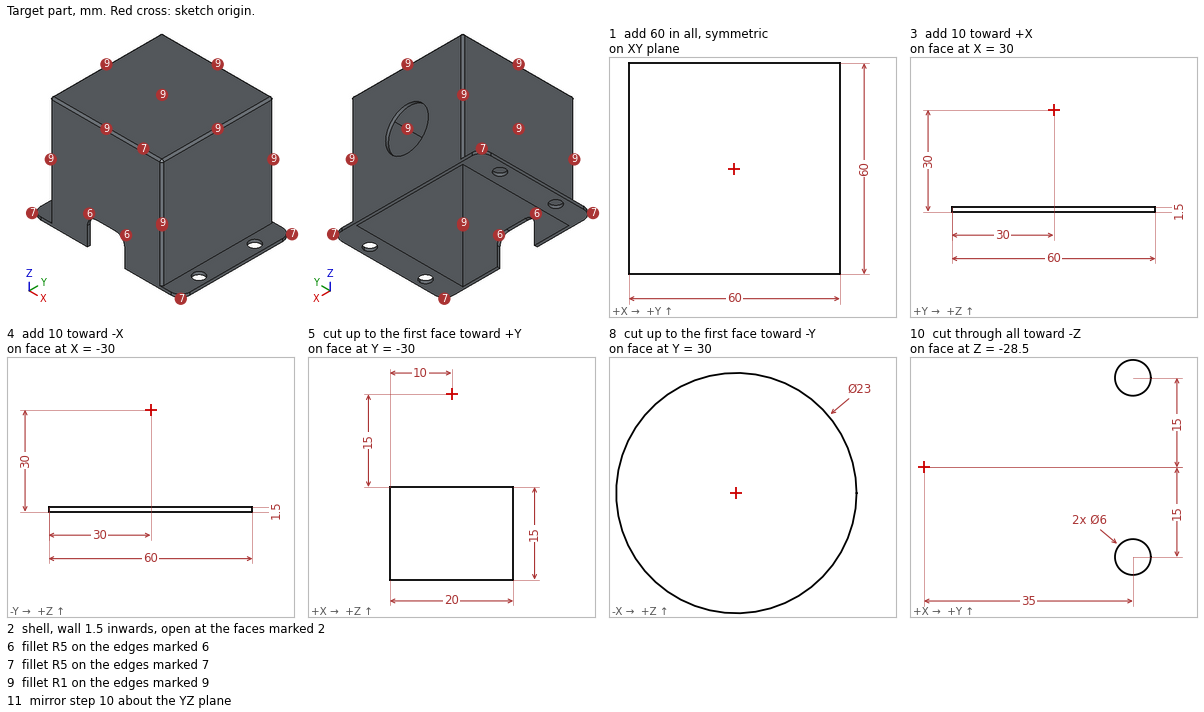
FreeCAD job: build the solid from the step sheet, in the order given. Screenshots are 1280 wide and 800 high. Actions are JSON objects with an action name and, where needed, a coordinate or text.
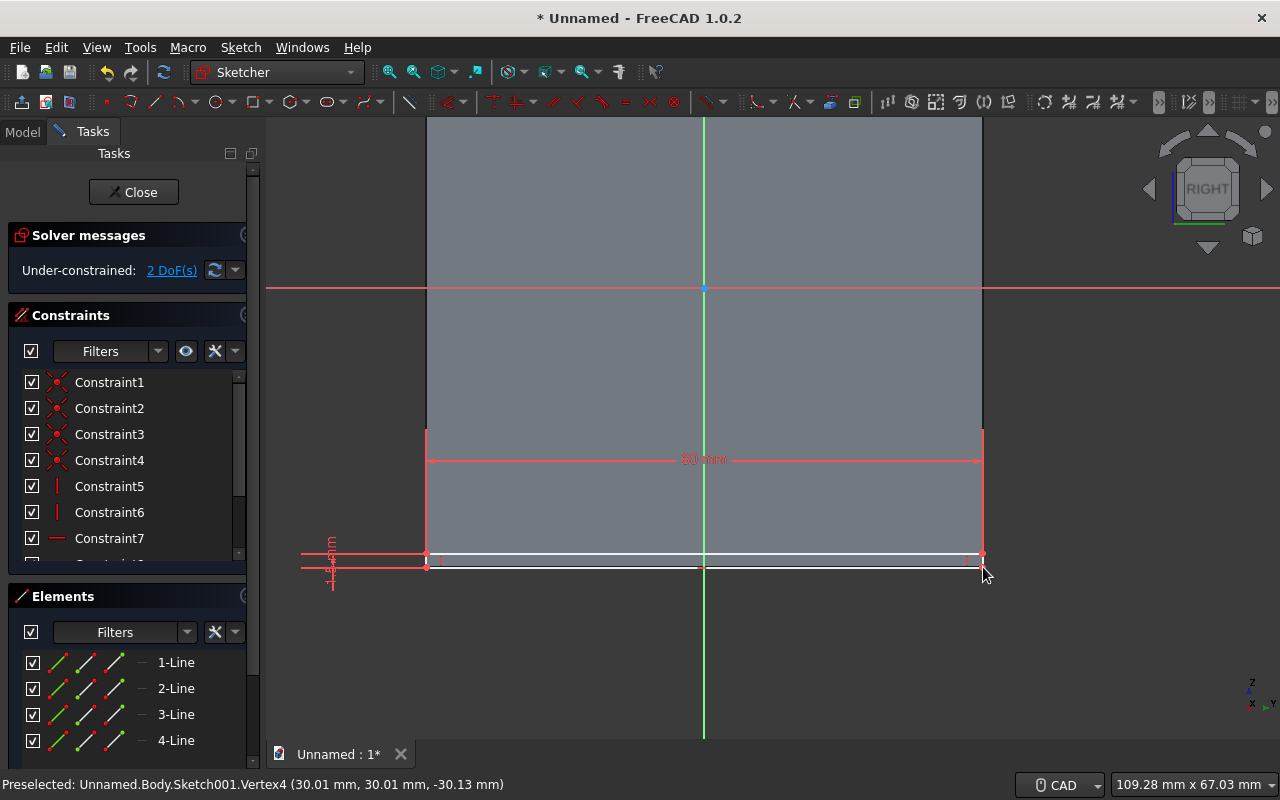
{"action": "left_click", "coordinate": [426, 554]}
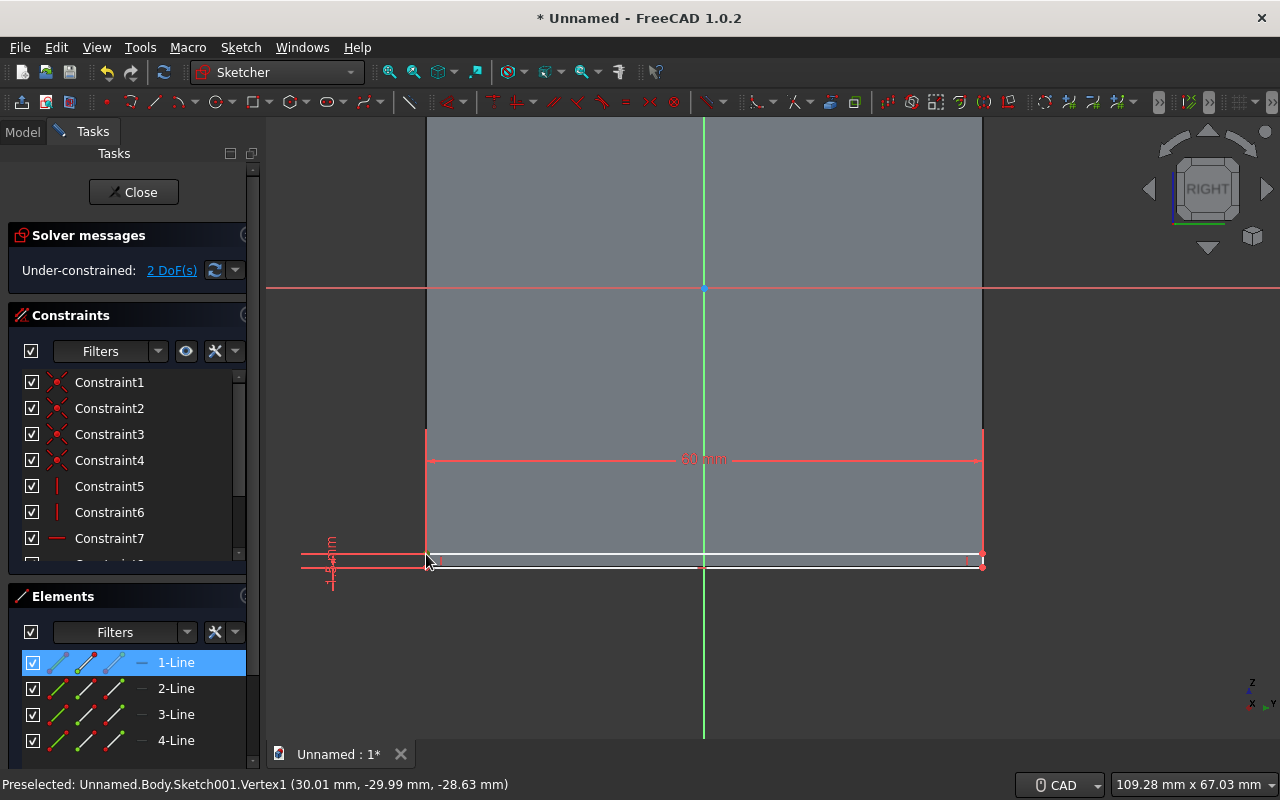
{"action": "key", "text": "l"}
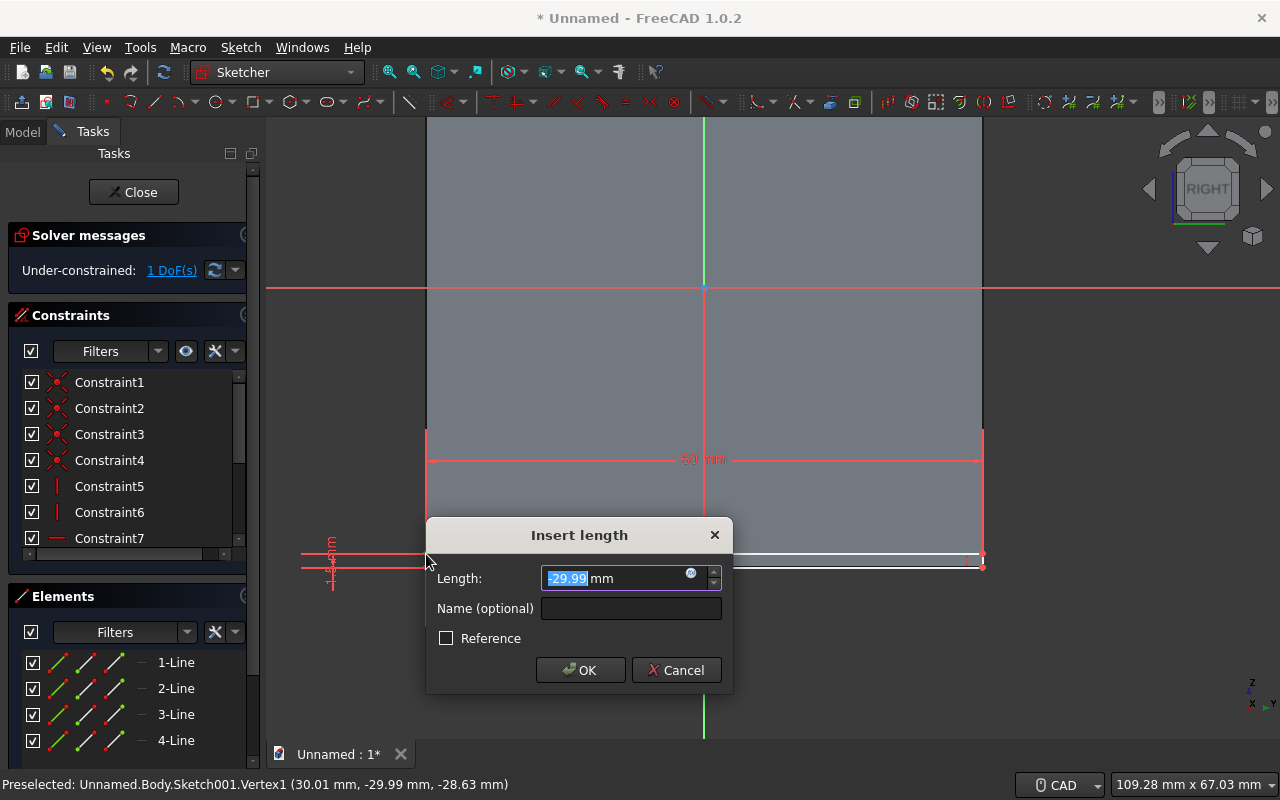
{"action": "type", "text": "-30"}
{"action": "key", "text": "Return"}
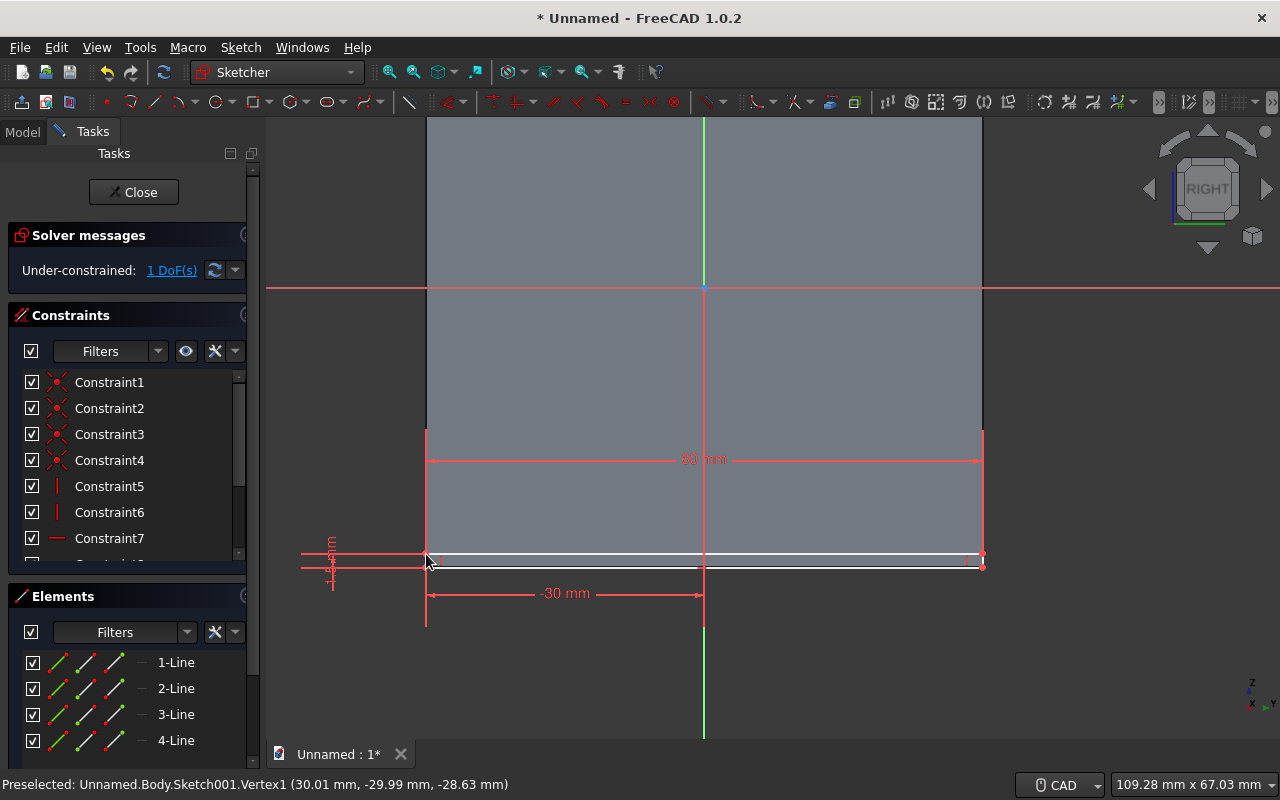
{"action": "left_click", "coordinate": [426, 568]}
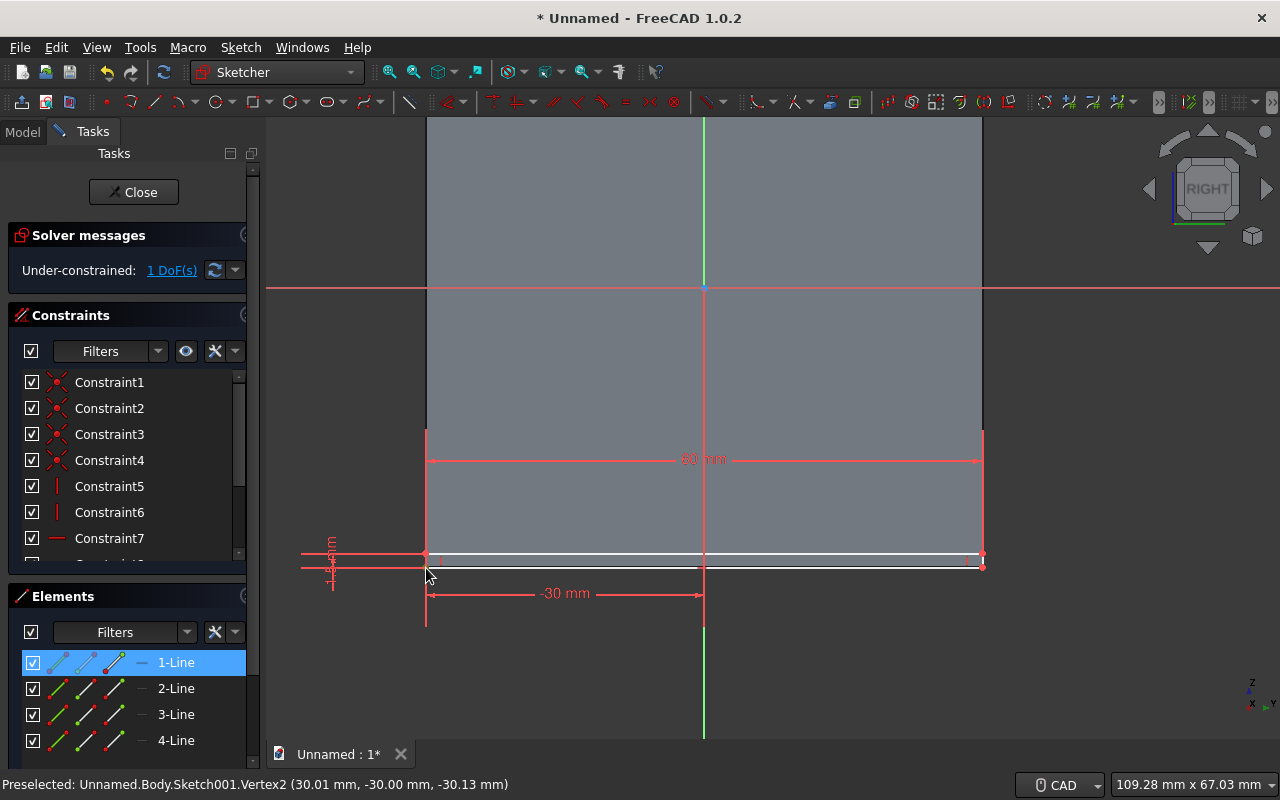
{"action": "key", "text": "i"}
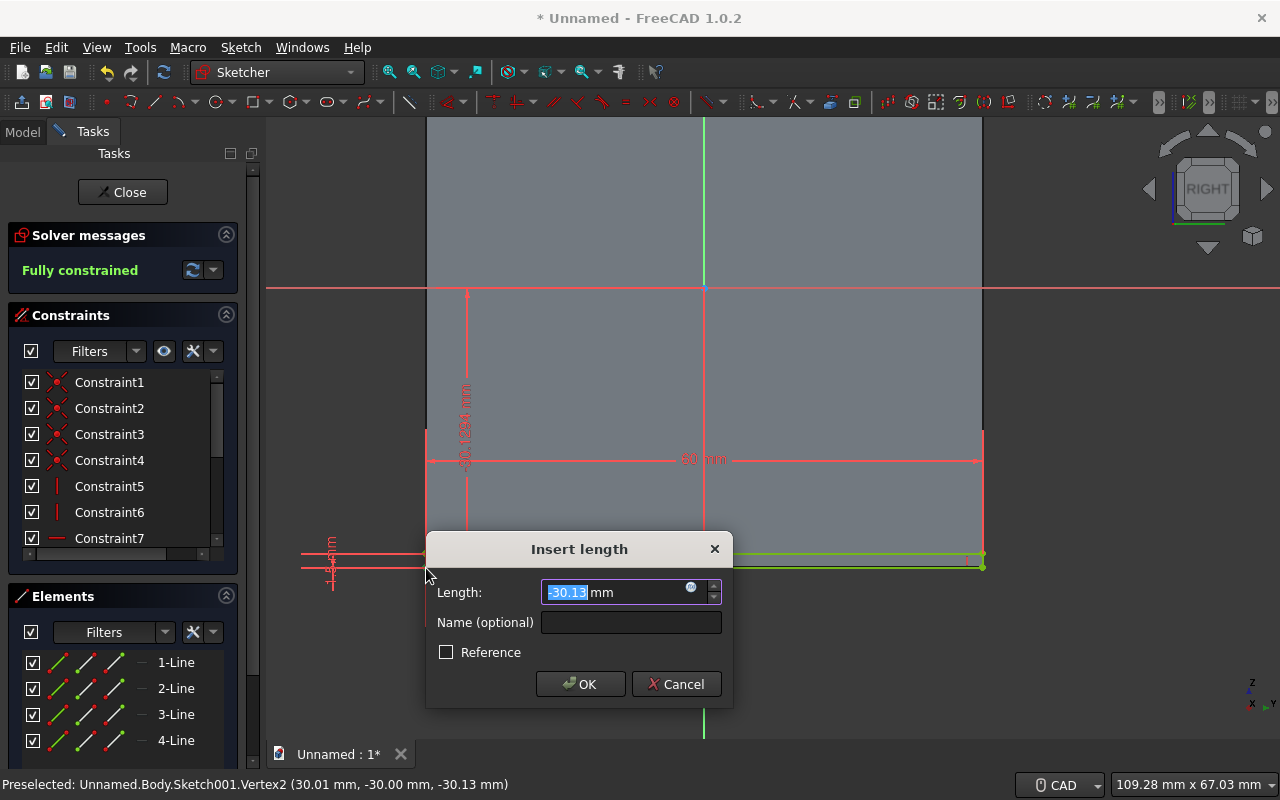
{"action": "type", "text": "-30"}
{"action": "key", "text": "Return"}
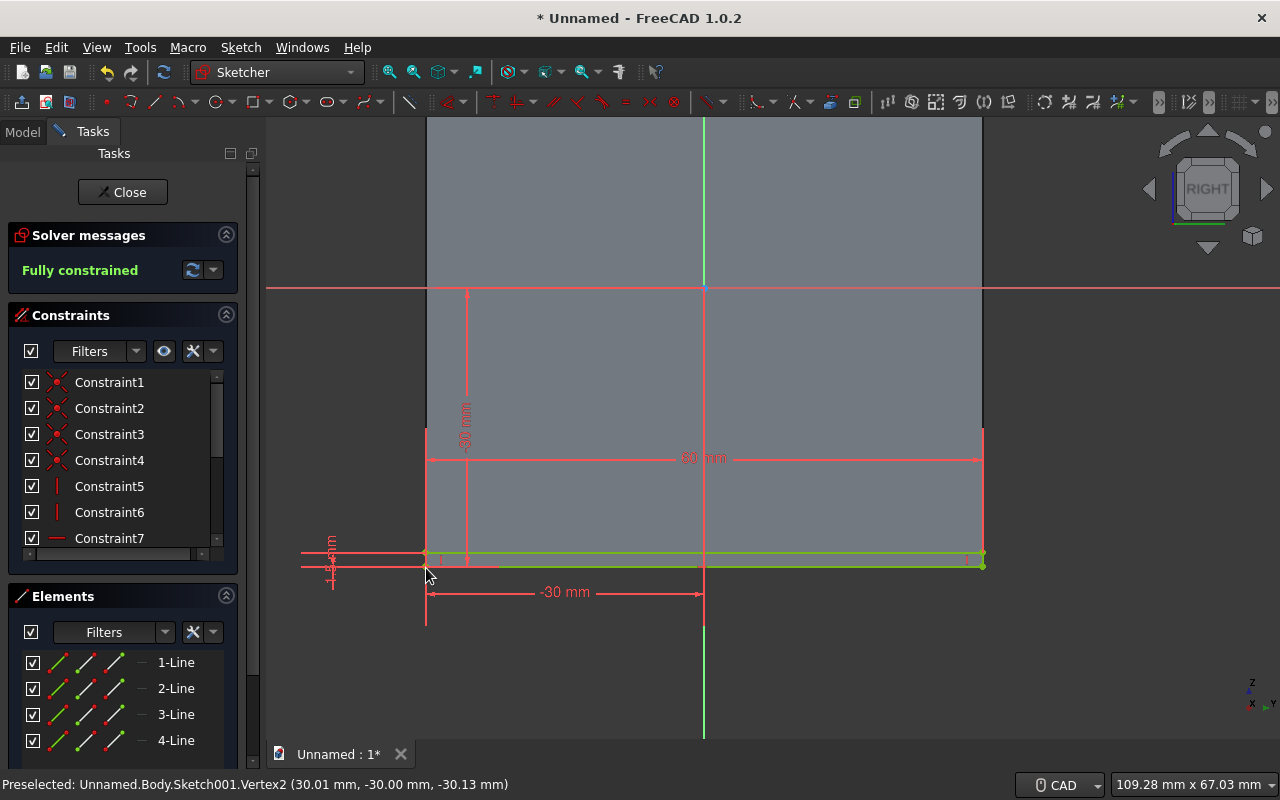
{"action": "left_click", "coordinate": [123, 192]}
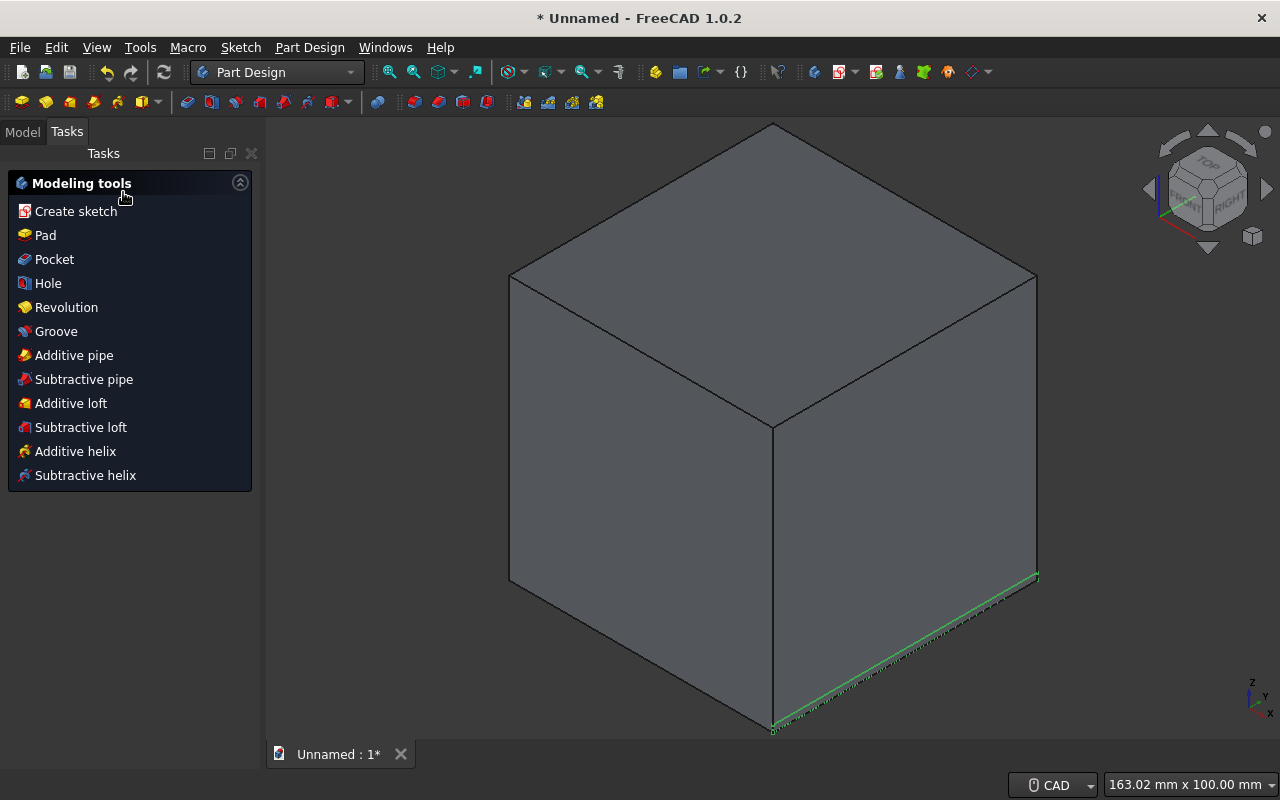
{"action": "left_click", "coordinate": [22, 102]}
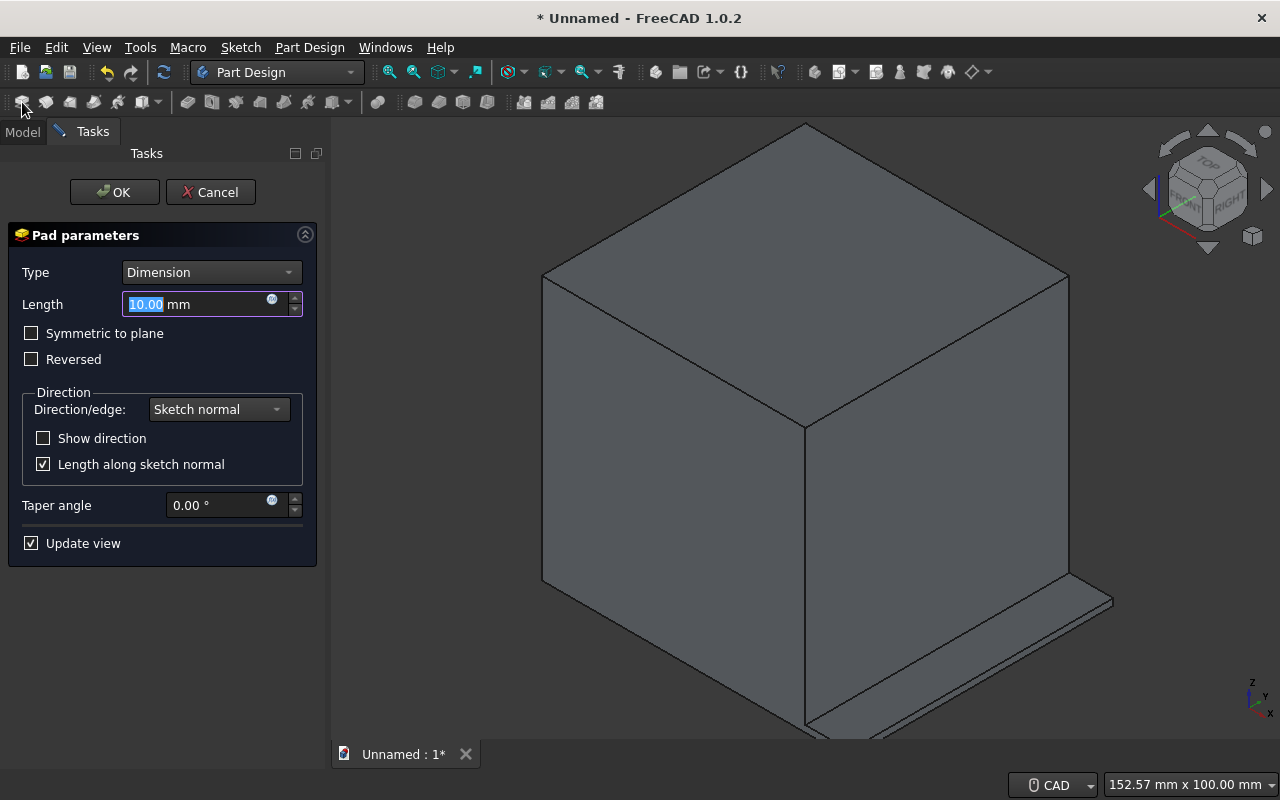
{"action": "type", "text": "10"}
{"action": "key", "text": "Tab"}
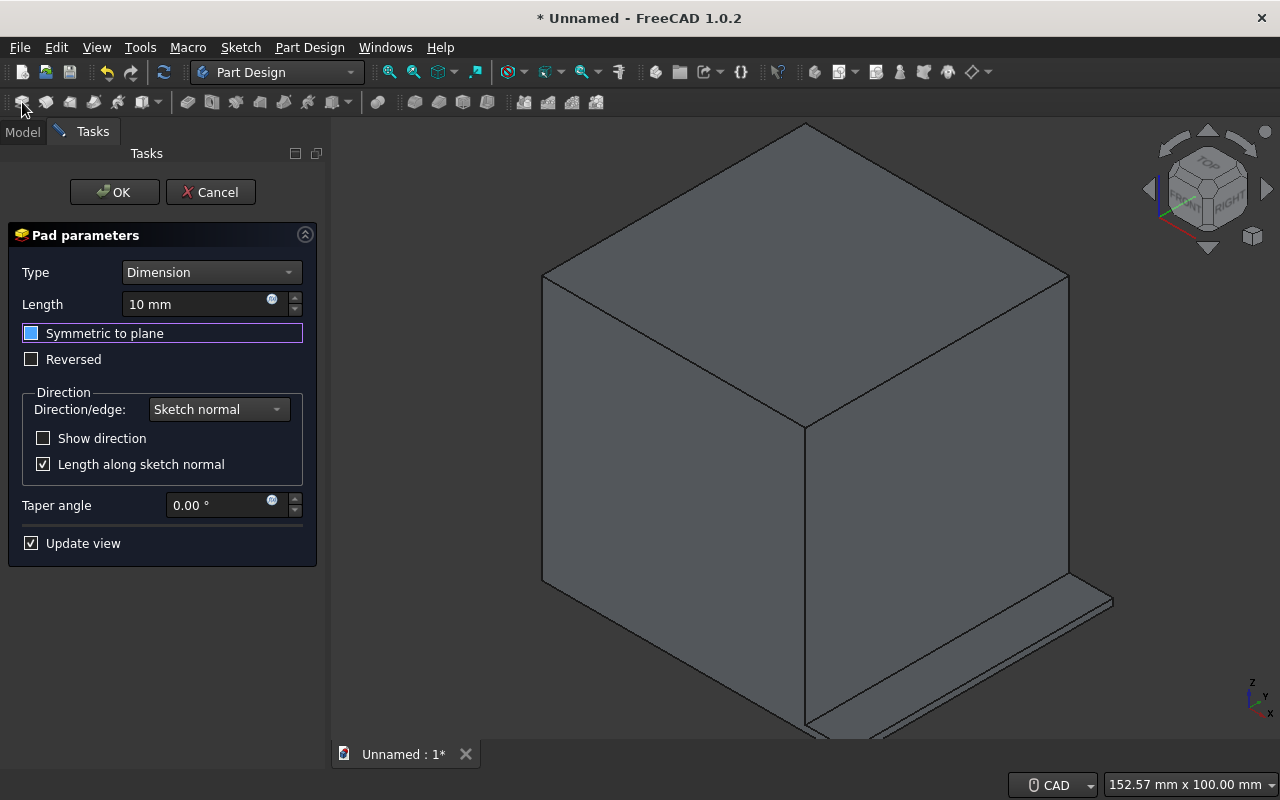
{"action": "left_click", "coordinate": [115, 192]}